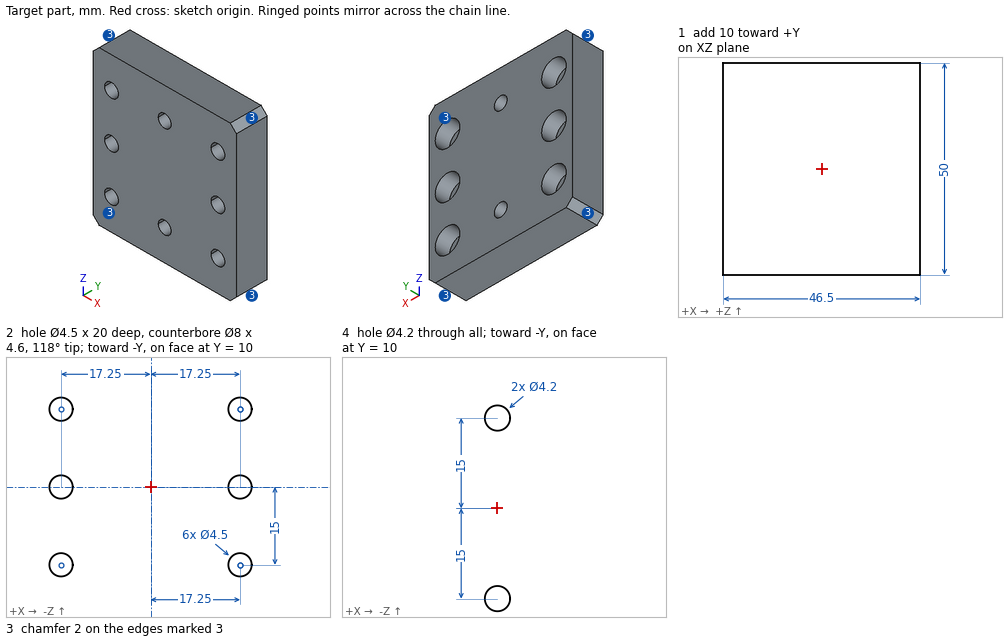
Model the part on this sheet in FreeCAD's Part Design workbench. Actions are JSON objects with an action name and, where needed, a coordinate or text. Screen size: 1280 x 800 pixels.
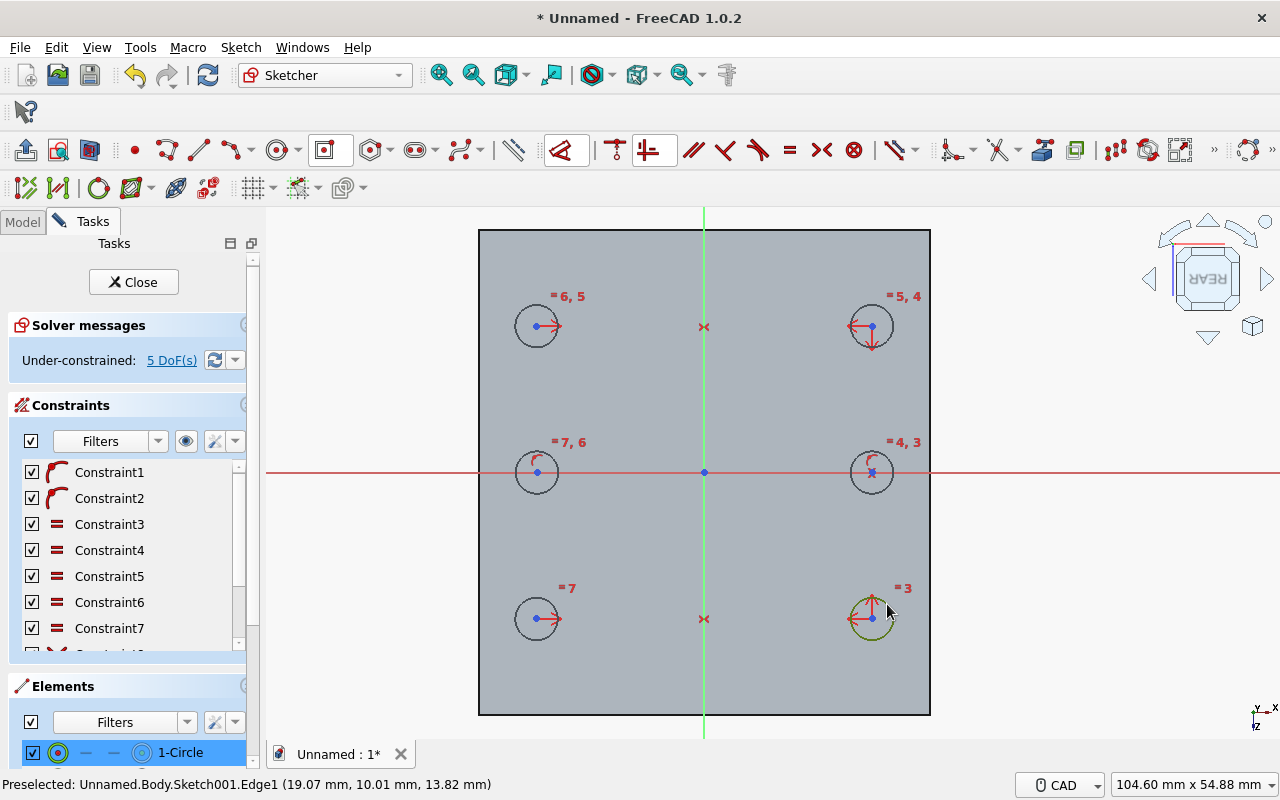
{"action": "key", "text": "k o"}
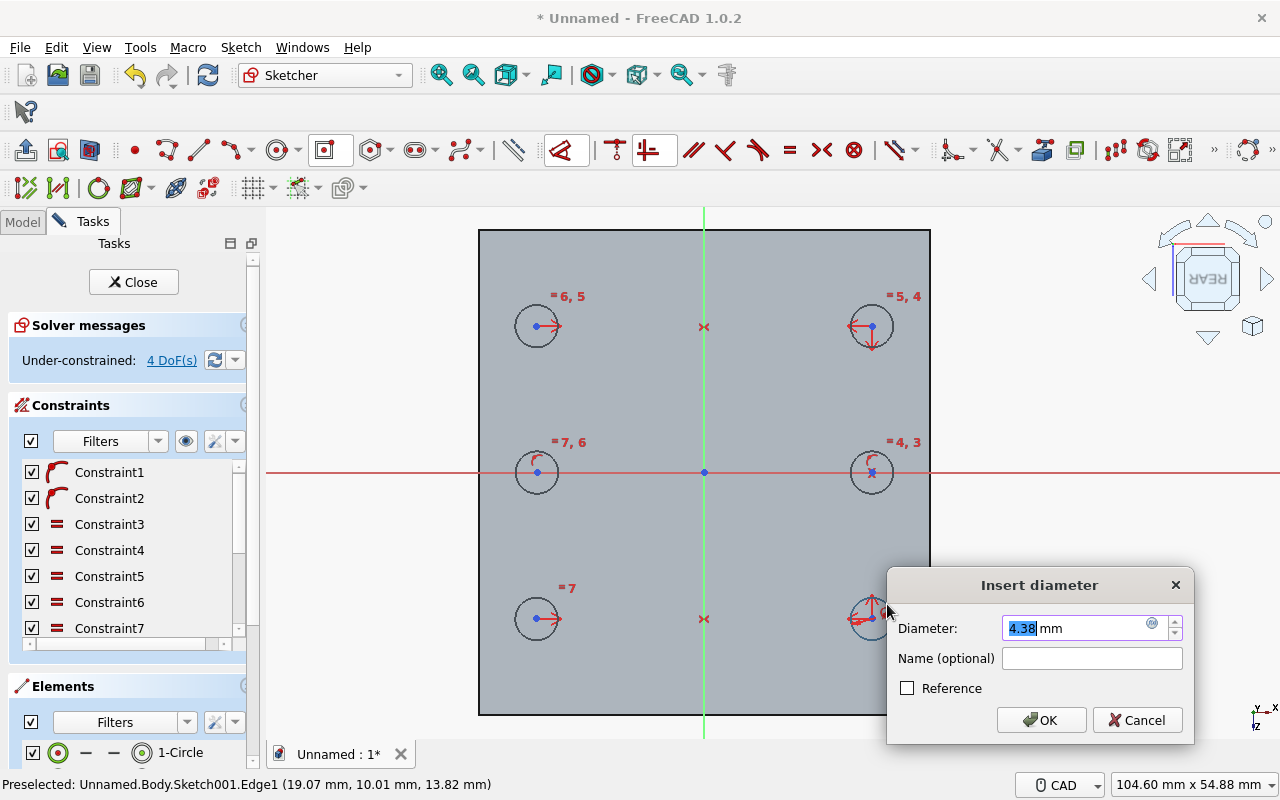
{"action": "type", "text": "4.5"}
{"action": "key", "text": "Return"}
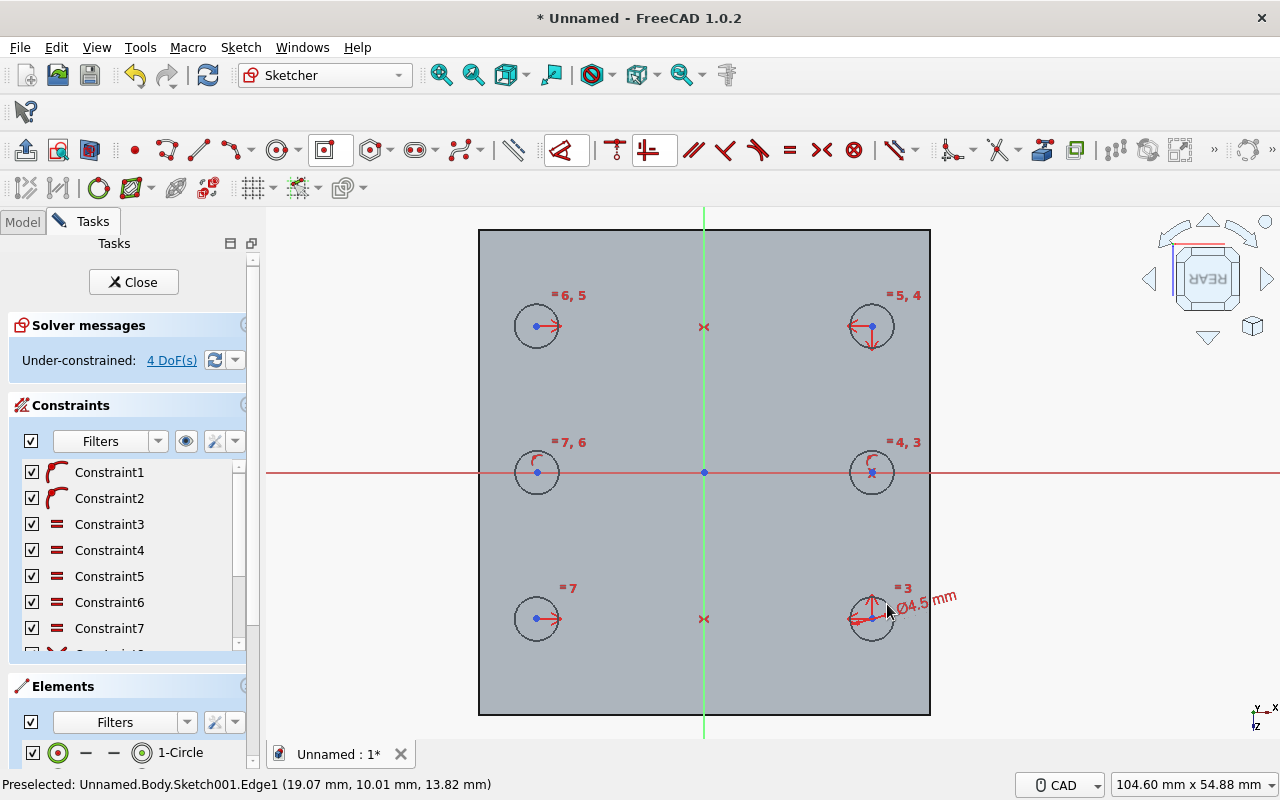
{"action": "left_click", "coordinate": [872, 619]}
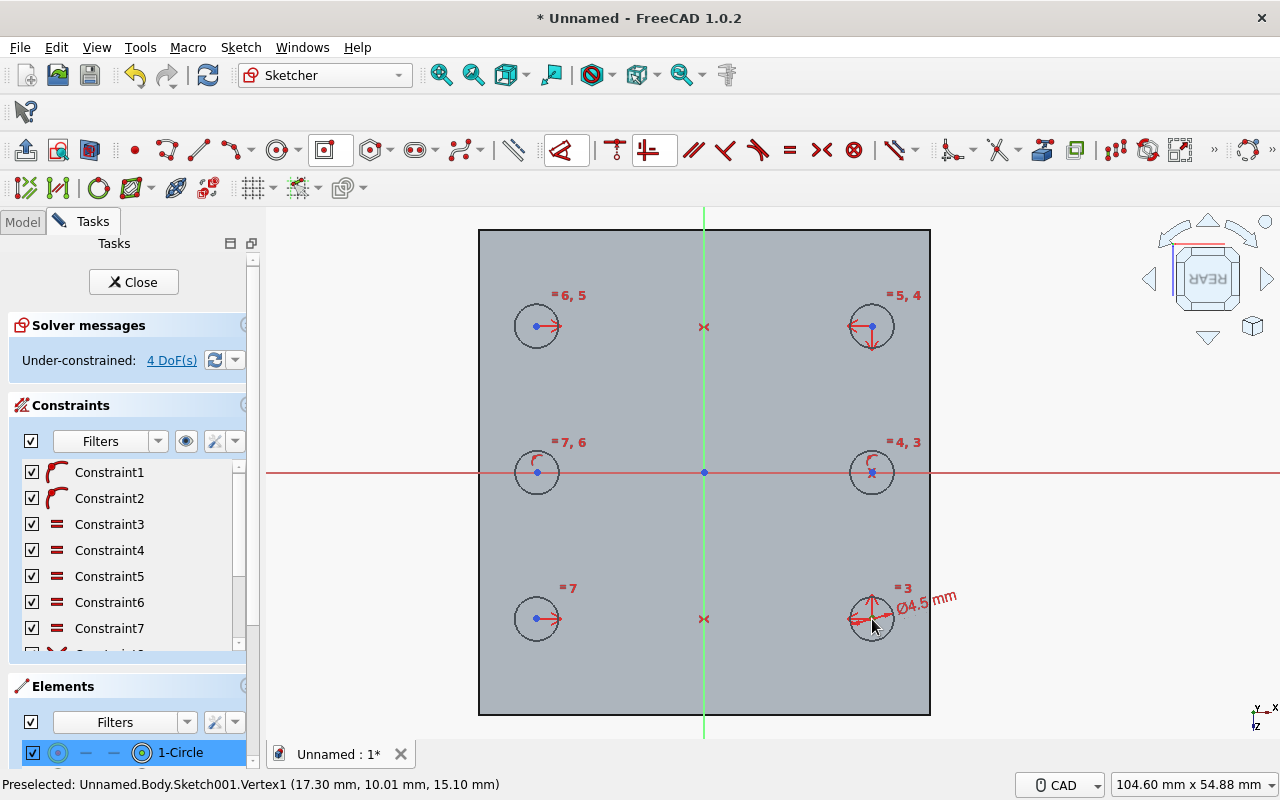
{"action": "key", "text": "i"}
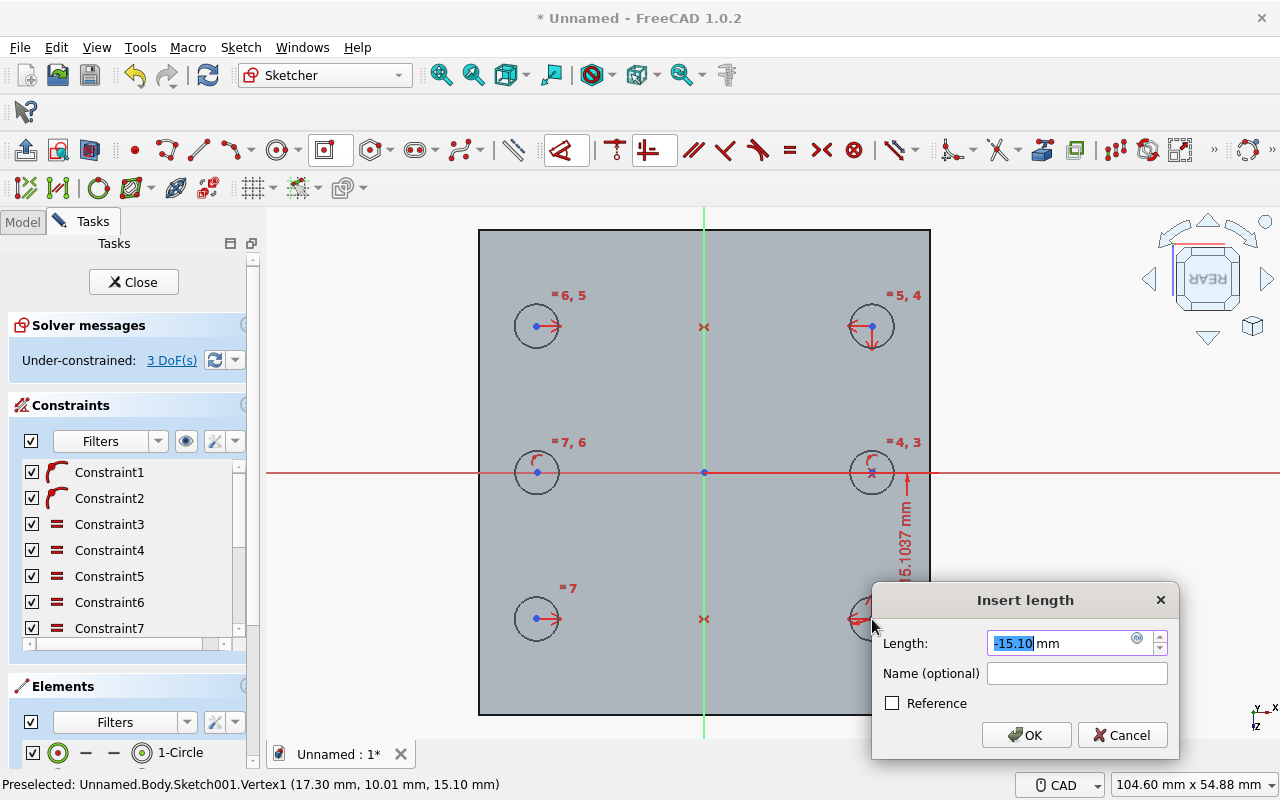
{"action": "type", "text": "-15"}
{"action": "key", "text": "Return"}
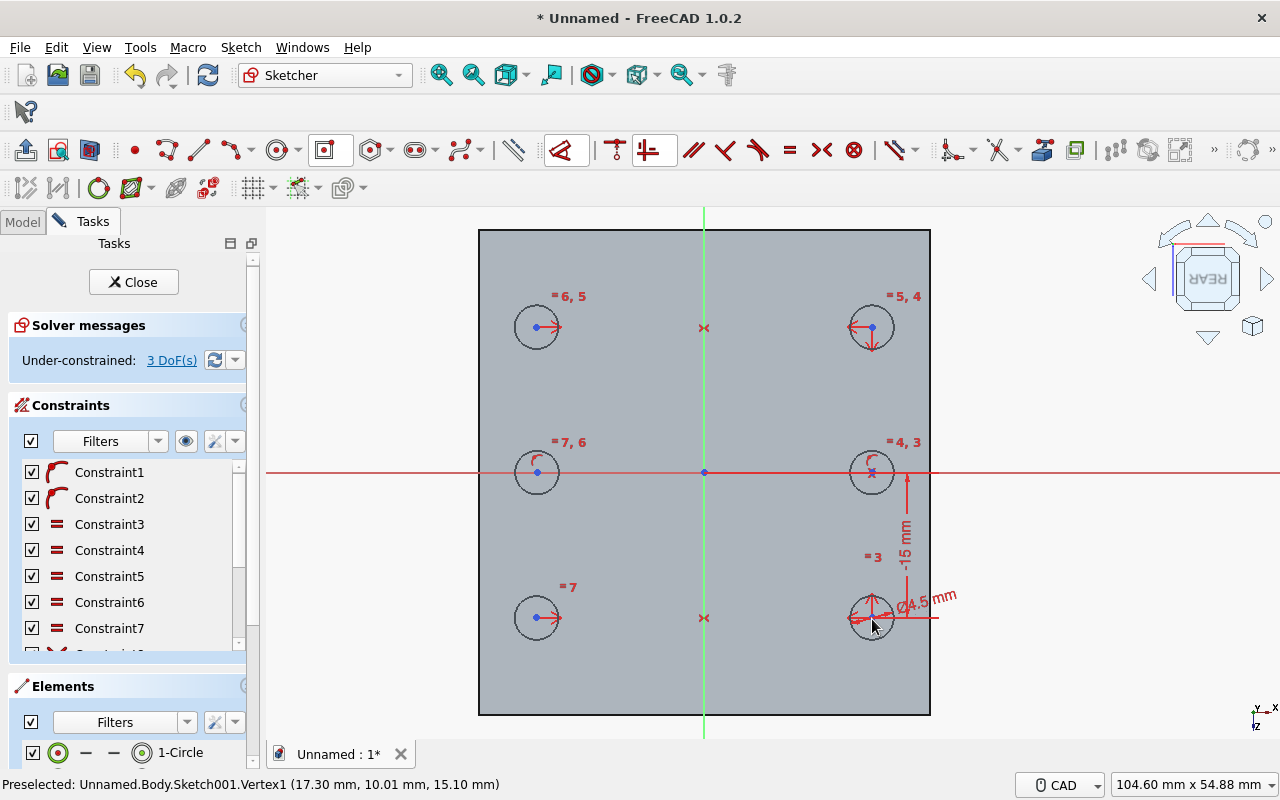
{"action": "left_click", "coordinate": [872, 618]}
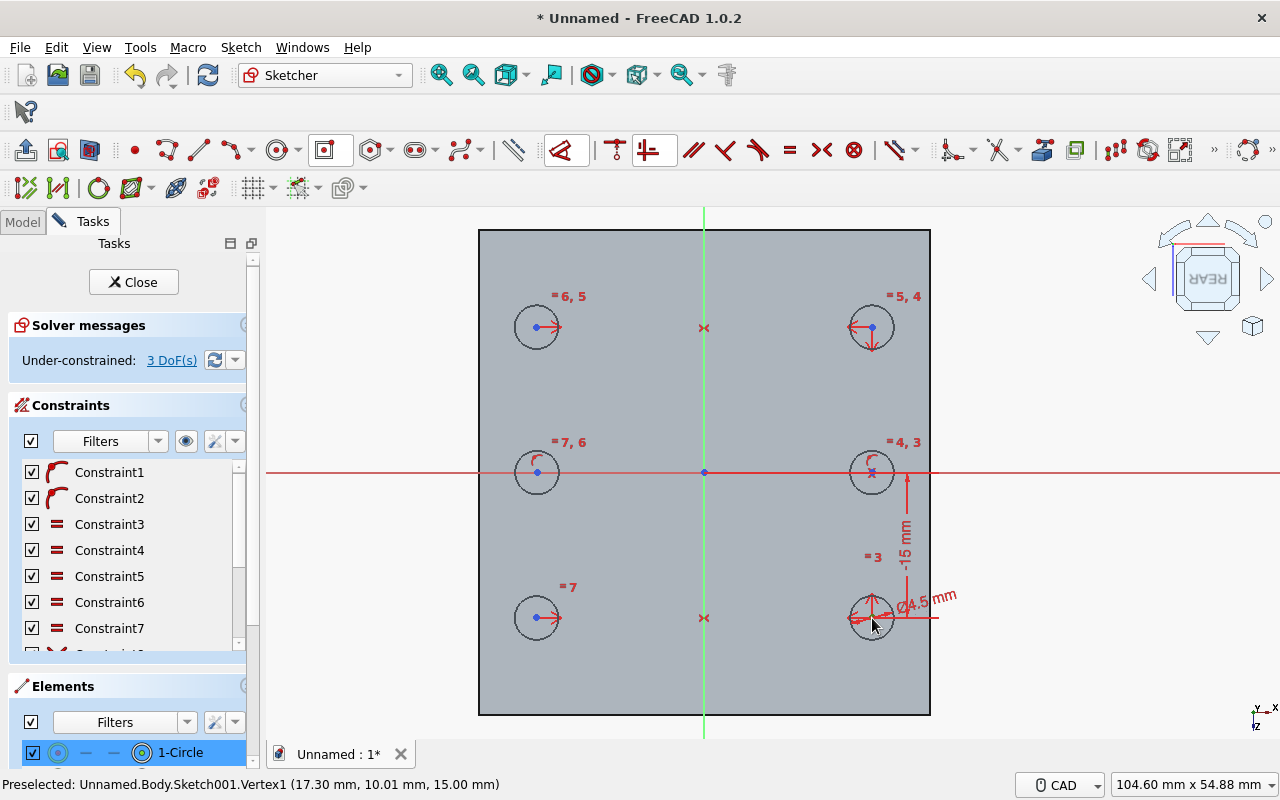
{"action": "left_click", "coordinate": [584, 150]}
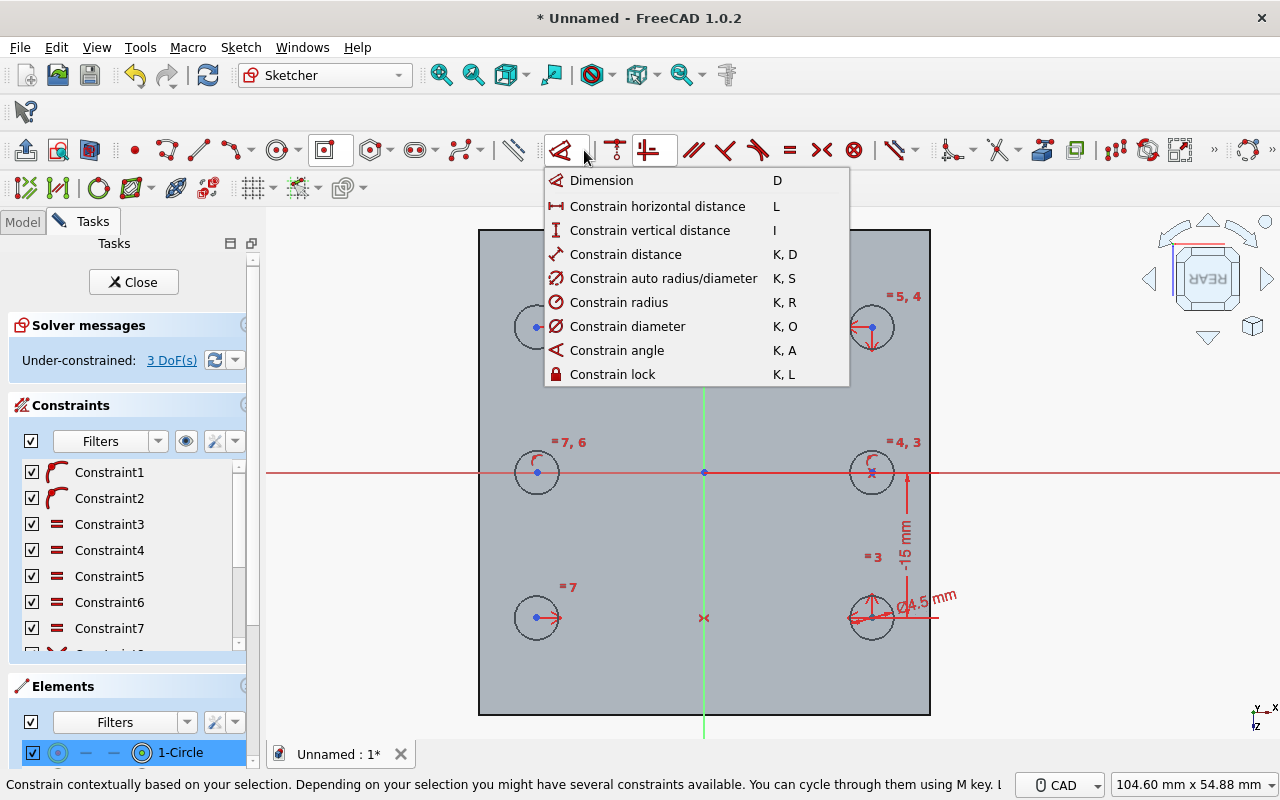
{"action": "left_click", "coordinate": [697, 206]}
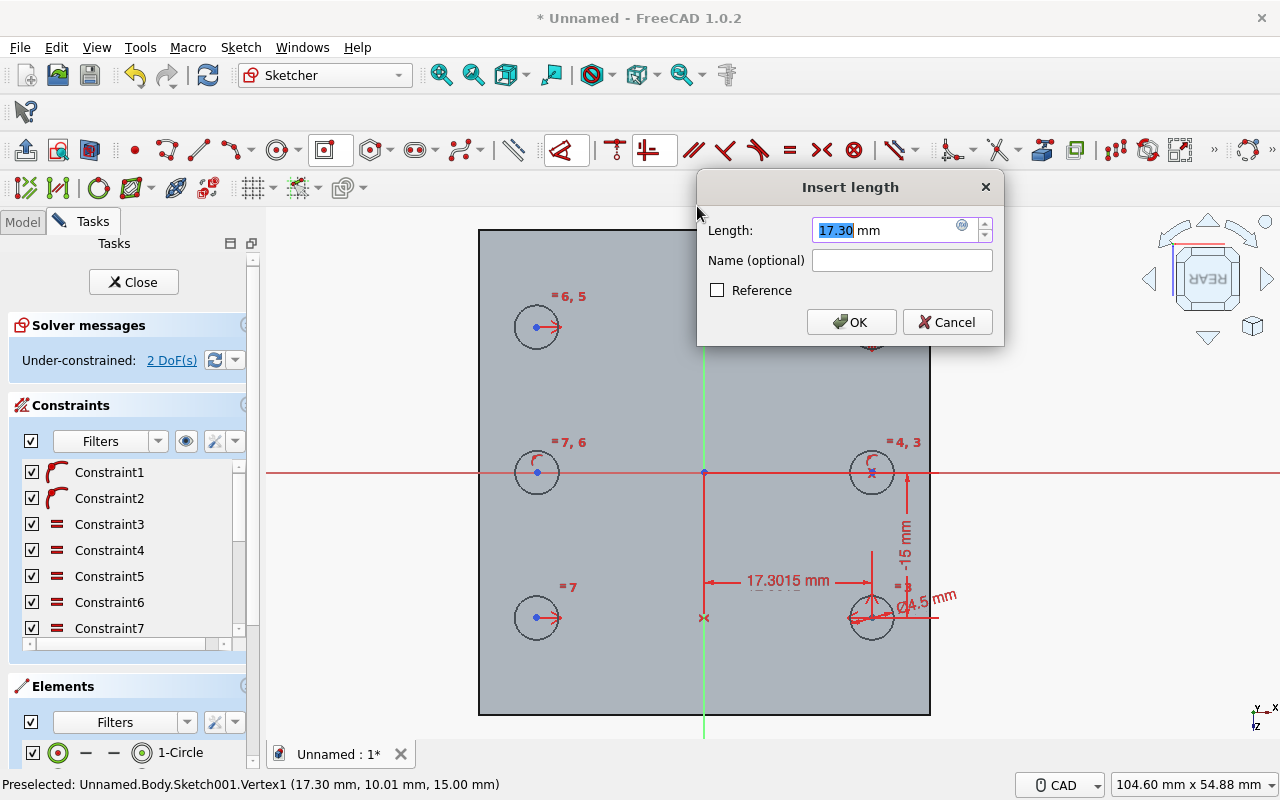
{"action": "type", "text": "17.25"}
{"action": "key", "text": "Return"}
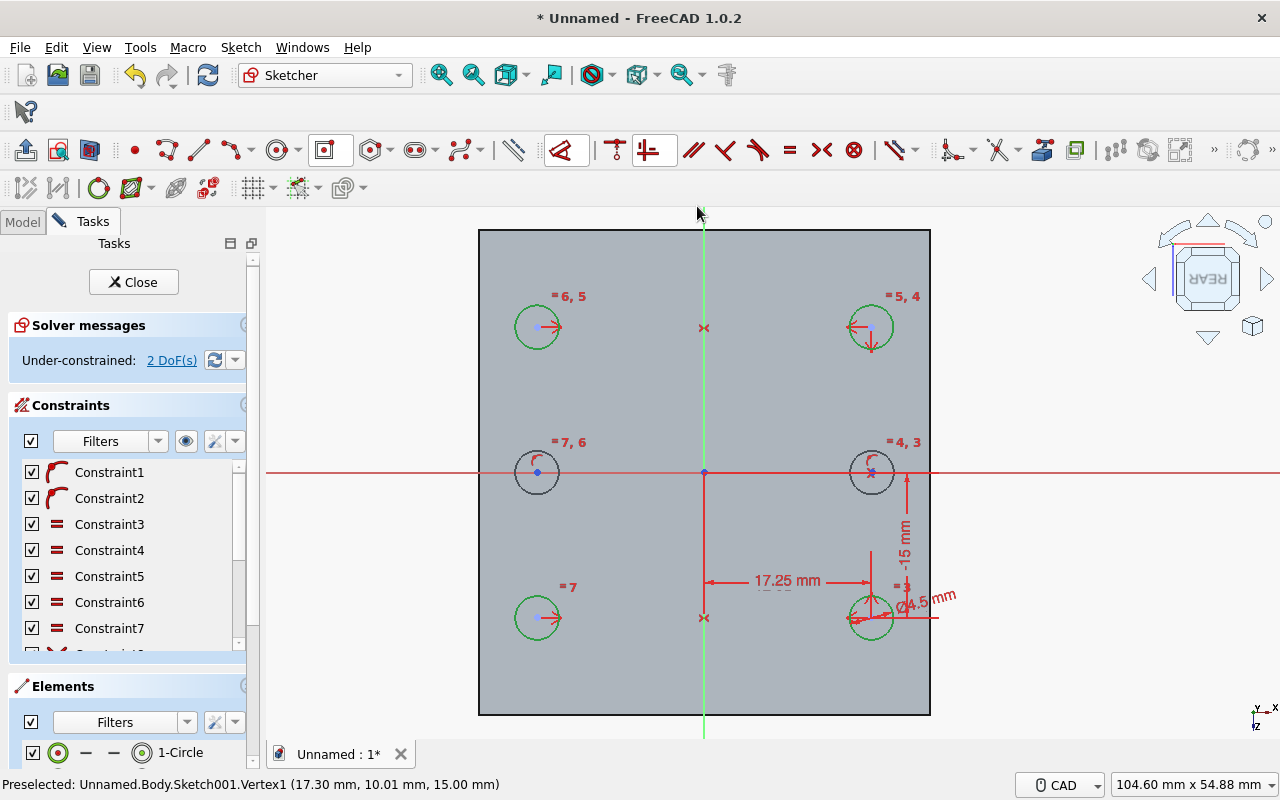
{"action": "left_click", "coordinate": [872, 473]}